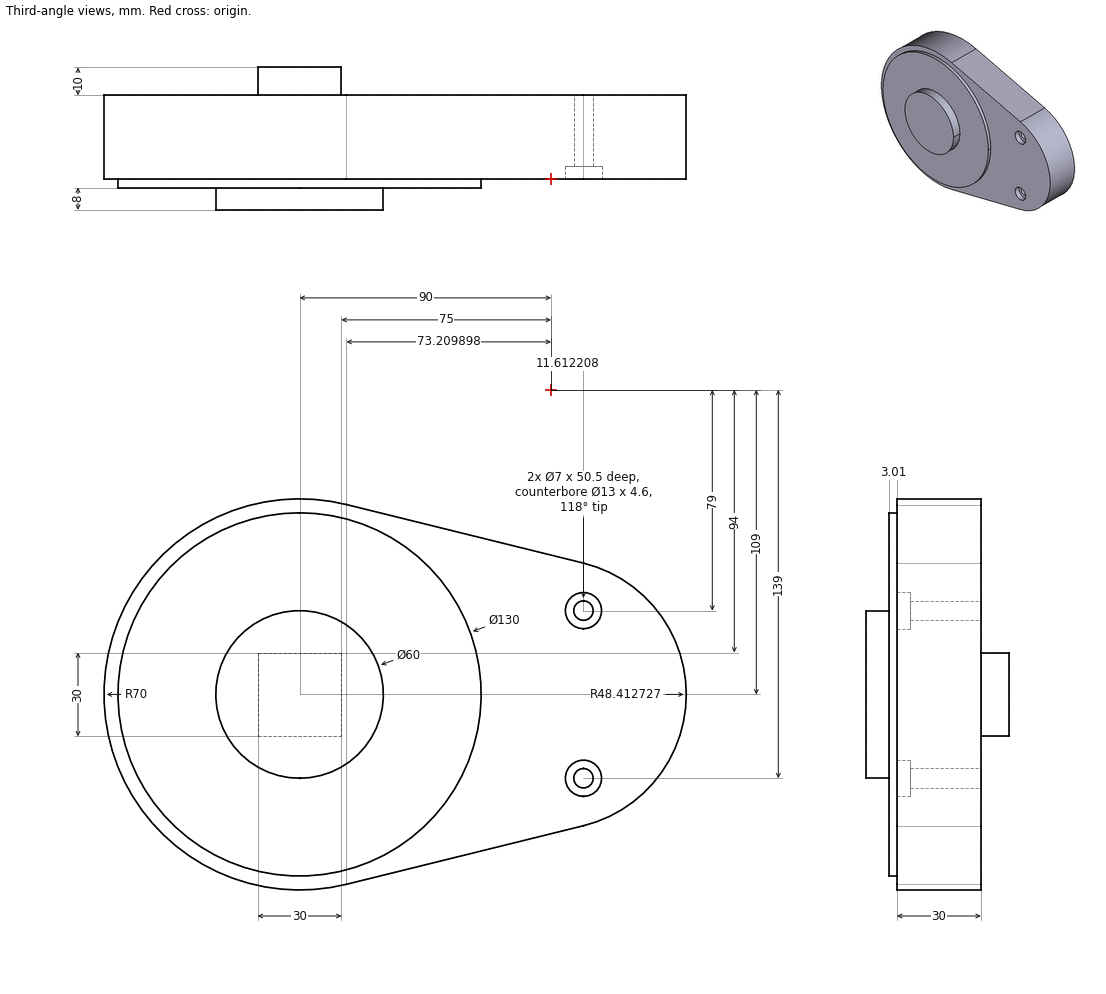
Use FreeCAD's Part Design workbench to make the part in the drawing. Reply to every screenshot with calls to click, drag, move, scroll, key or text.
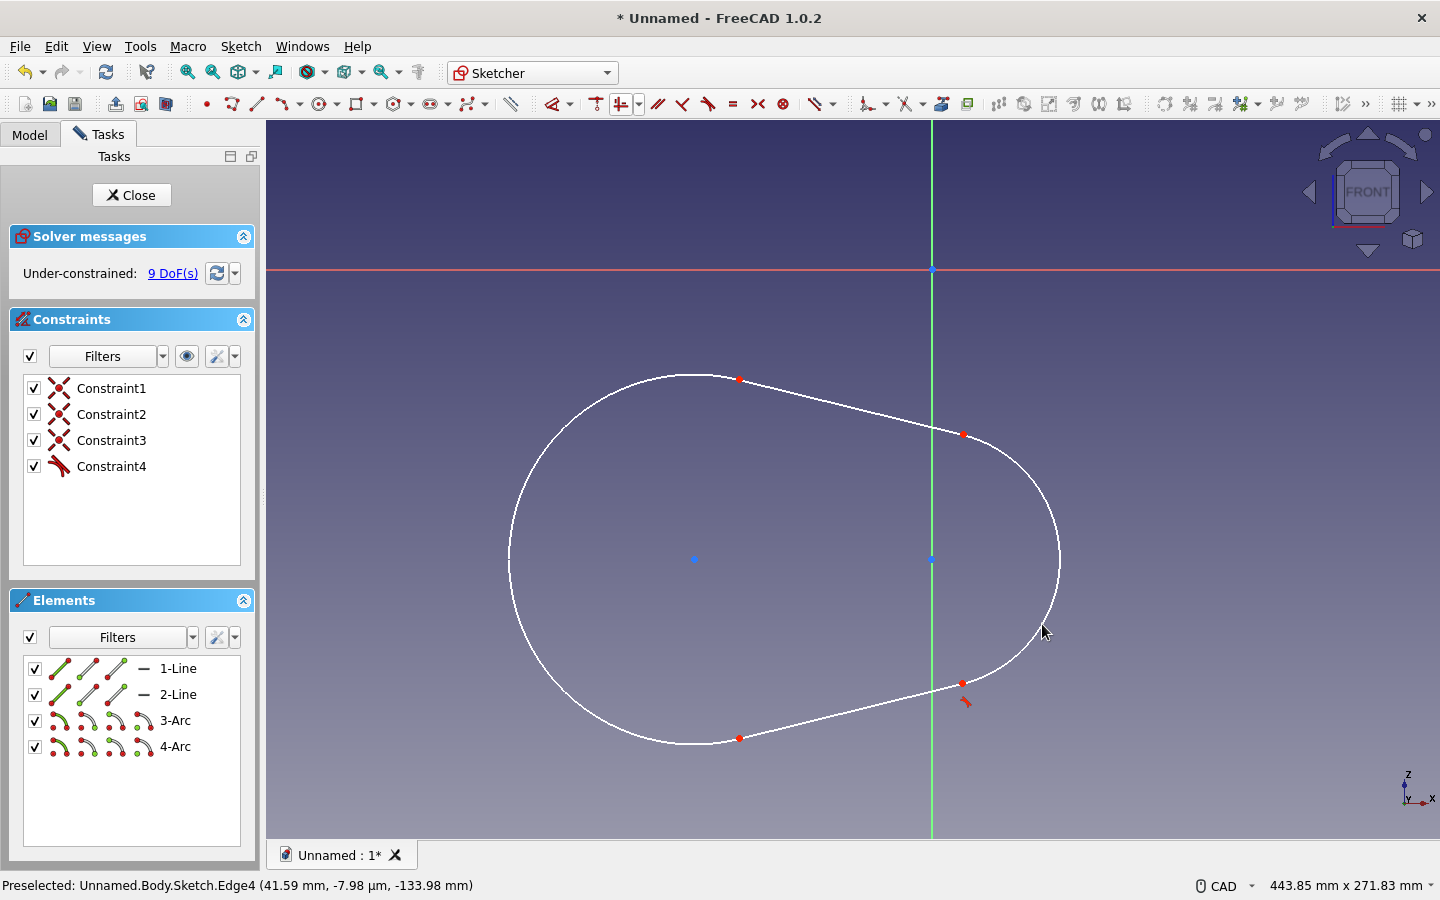
click(806, 397)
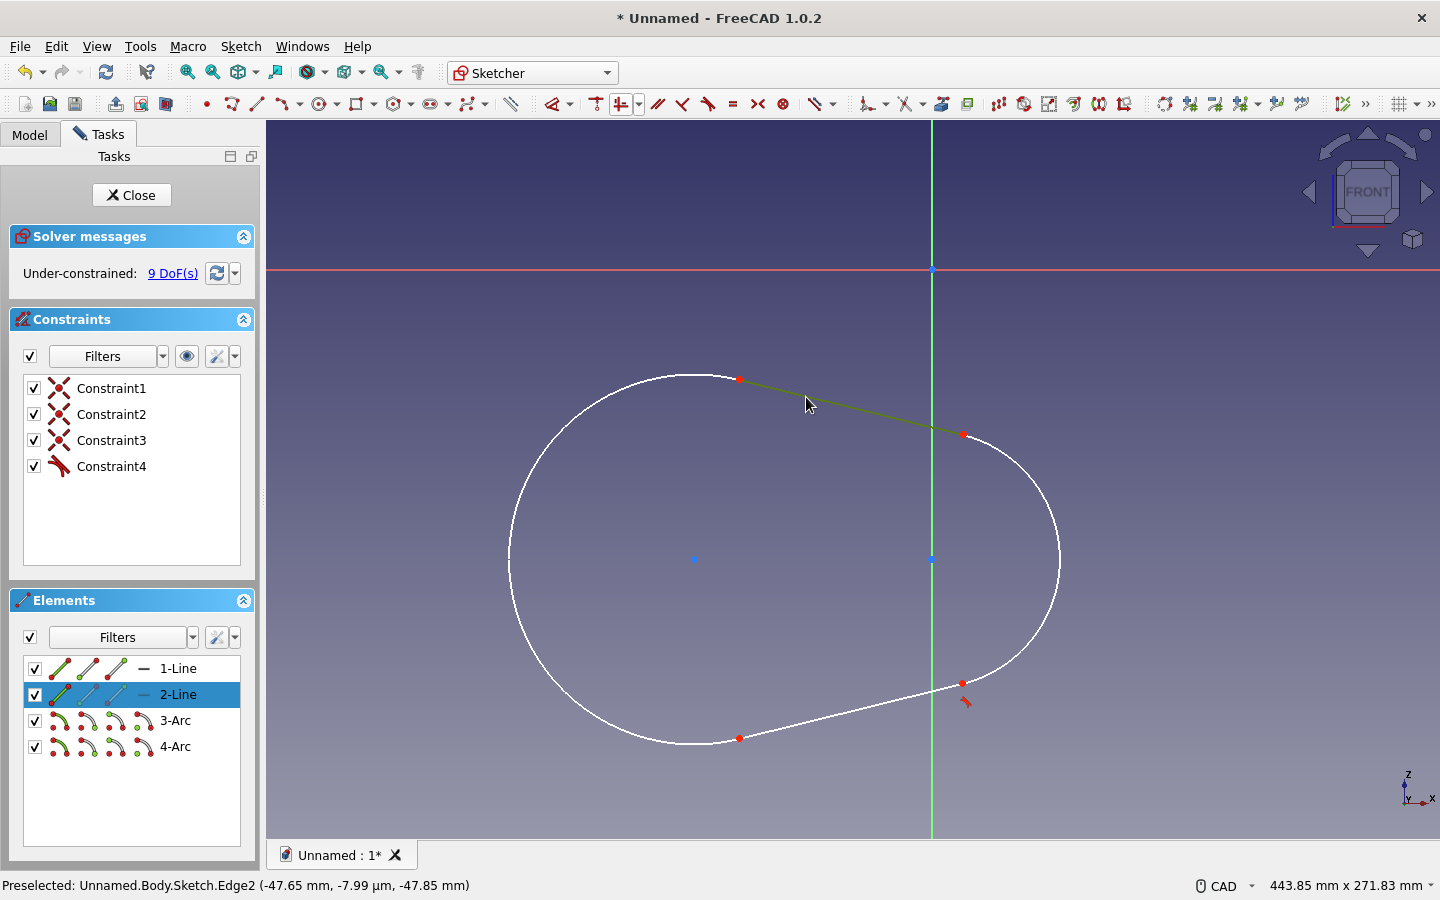
click(1042, 625)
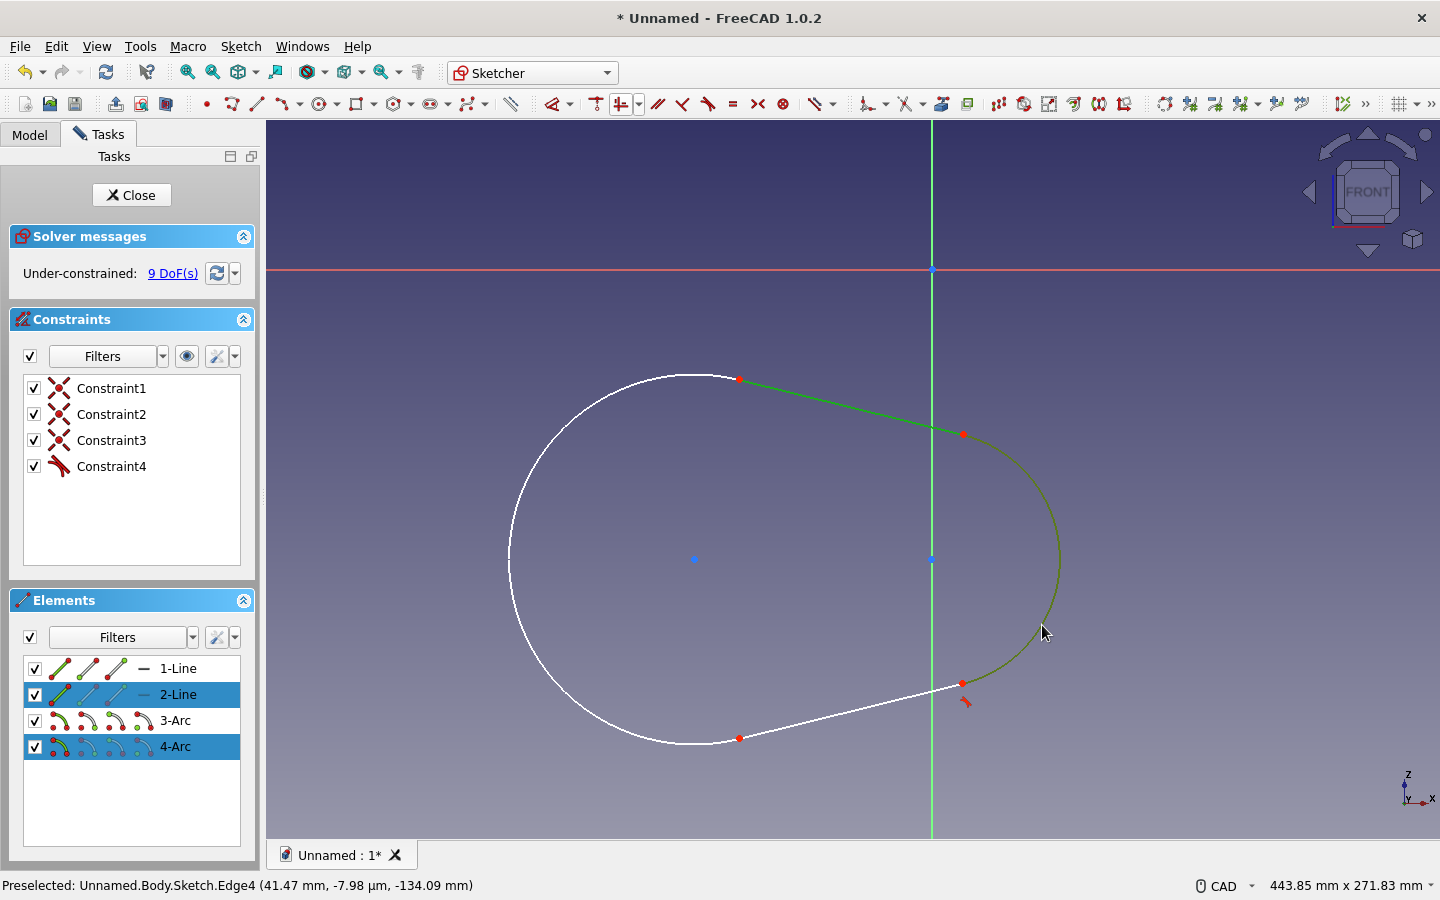
key(t)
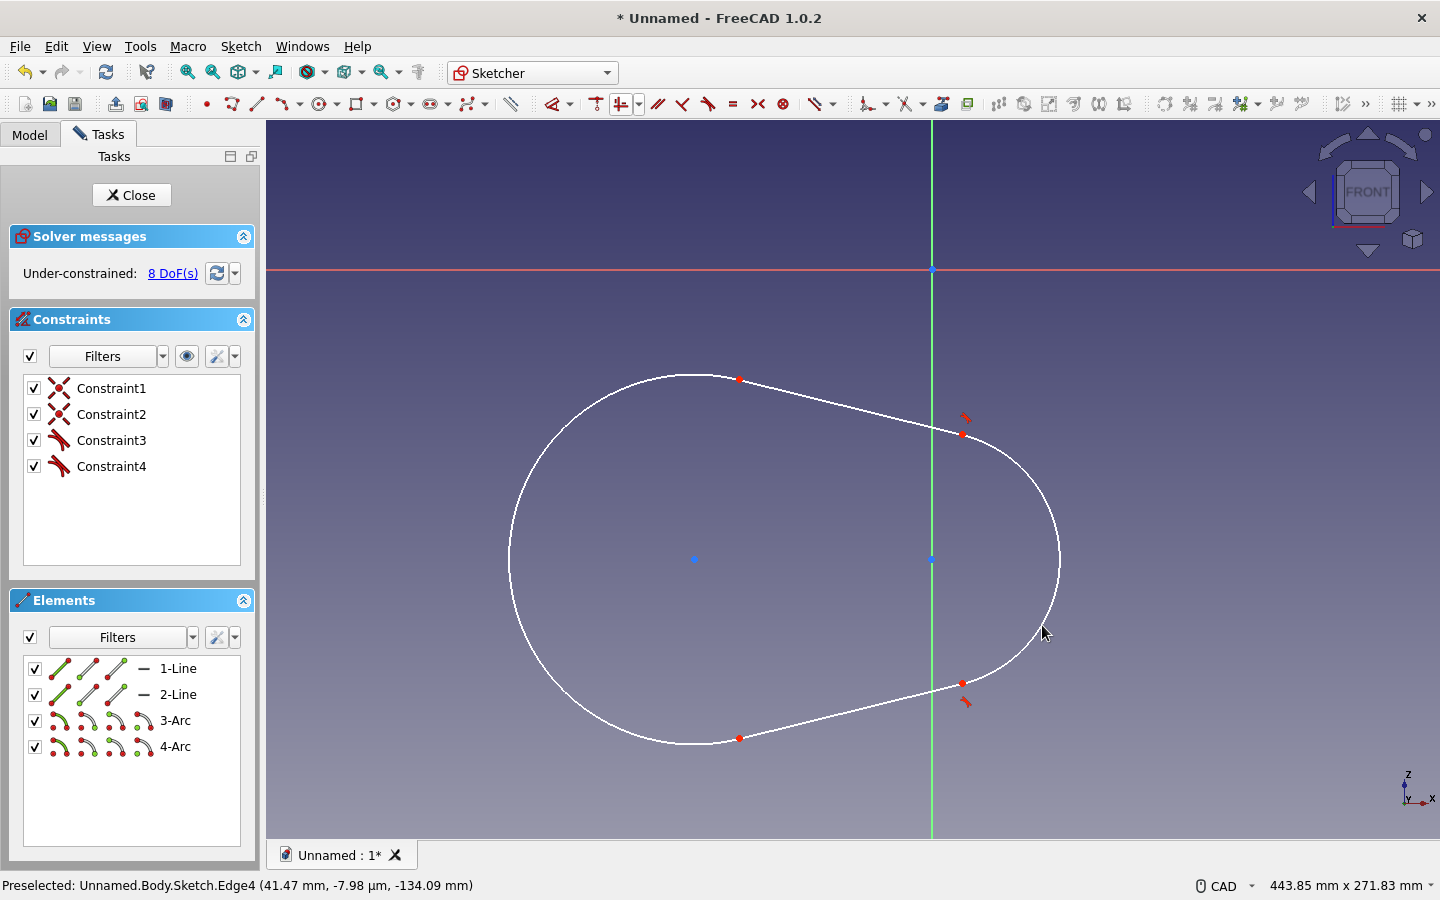
click(932, 560)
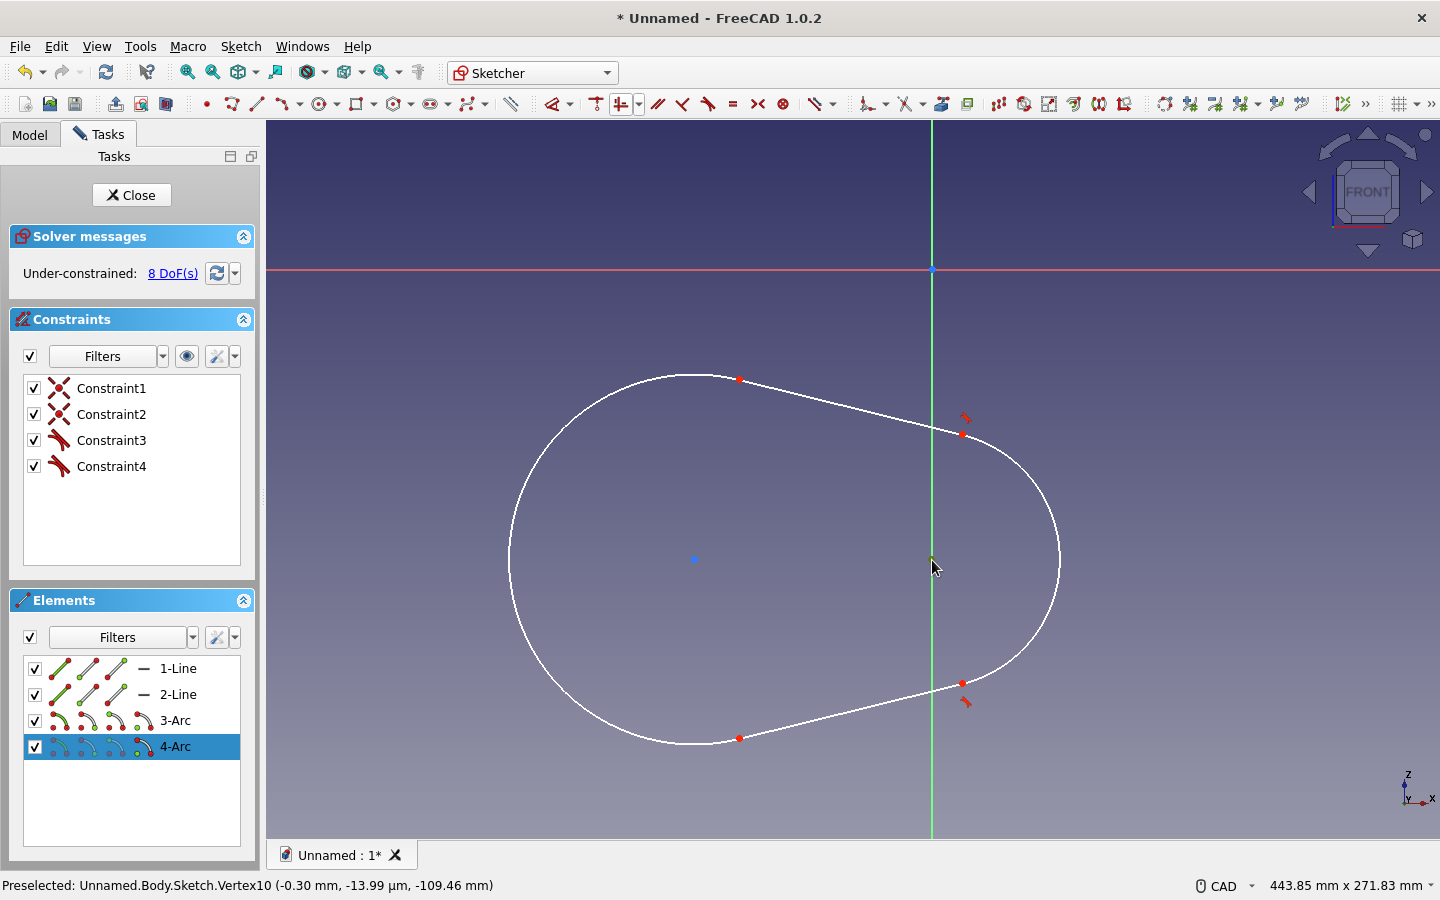
click(932, 764)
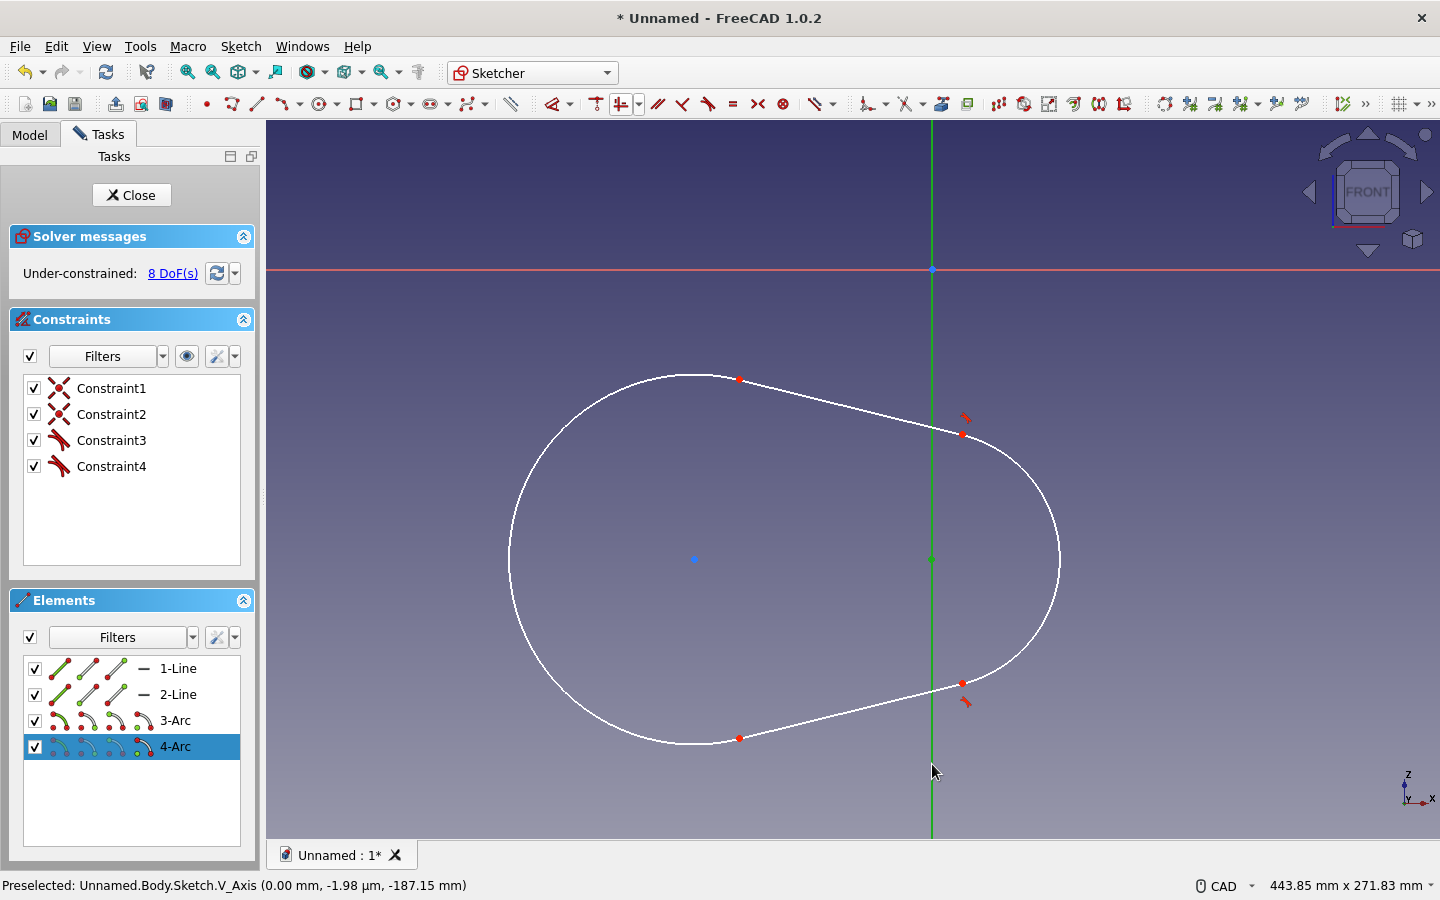
key(c)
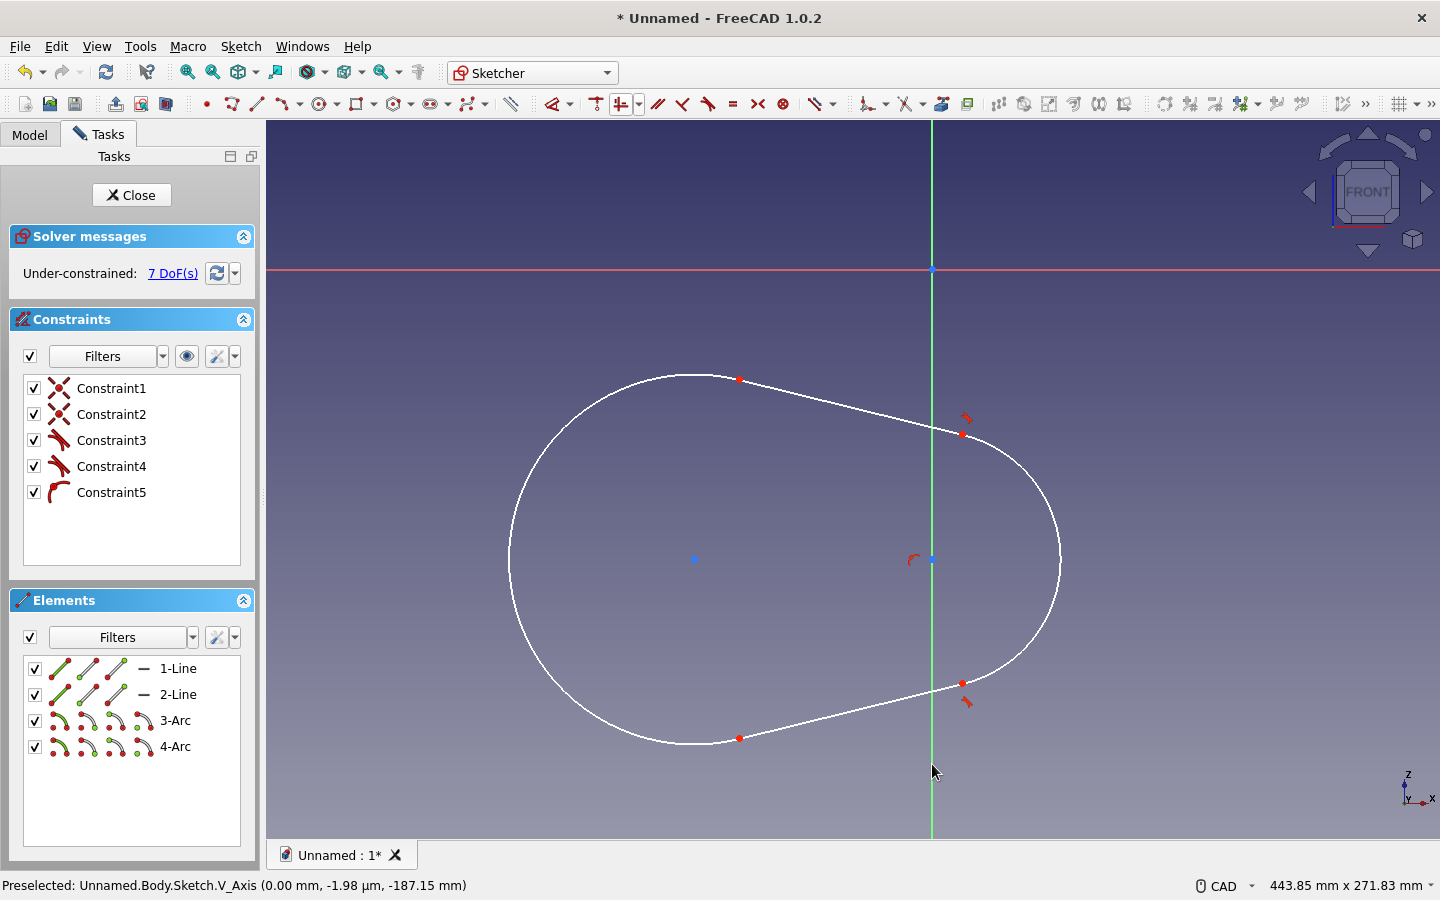
key(d)